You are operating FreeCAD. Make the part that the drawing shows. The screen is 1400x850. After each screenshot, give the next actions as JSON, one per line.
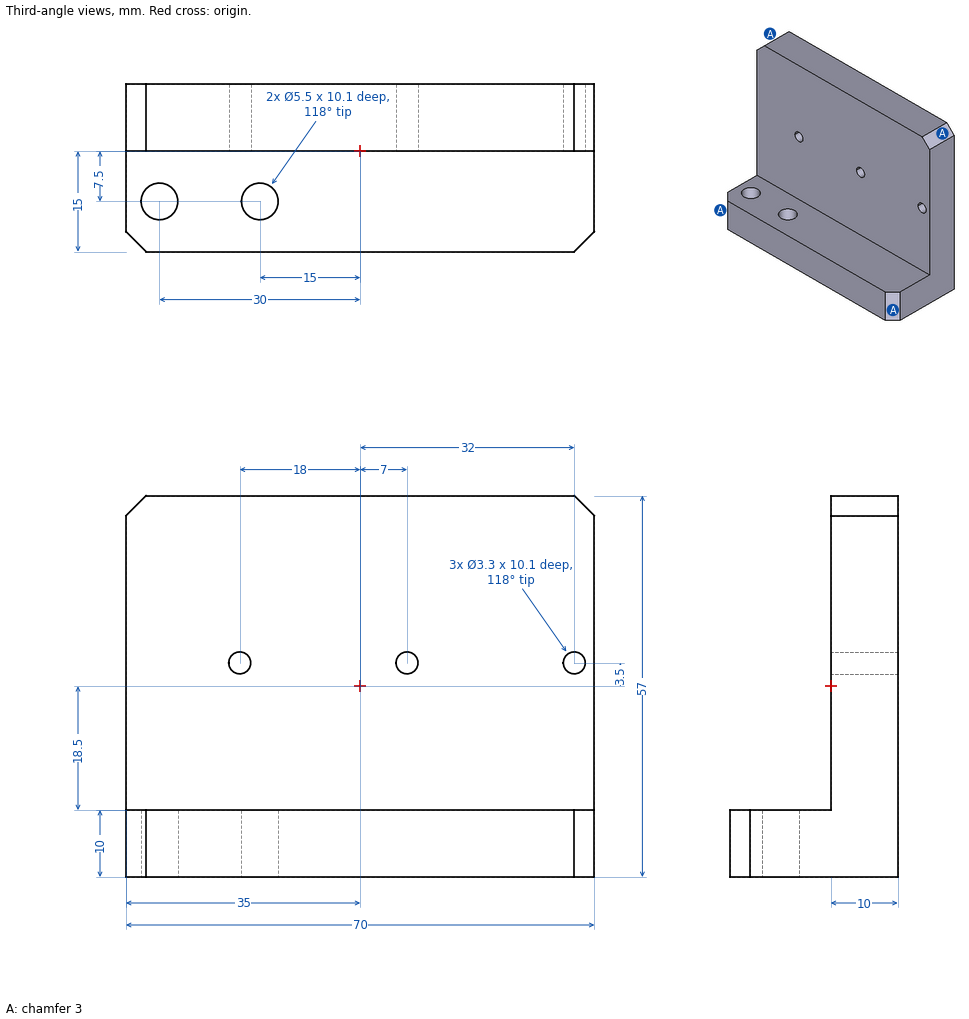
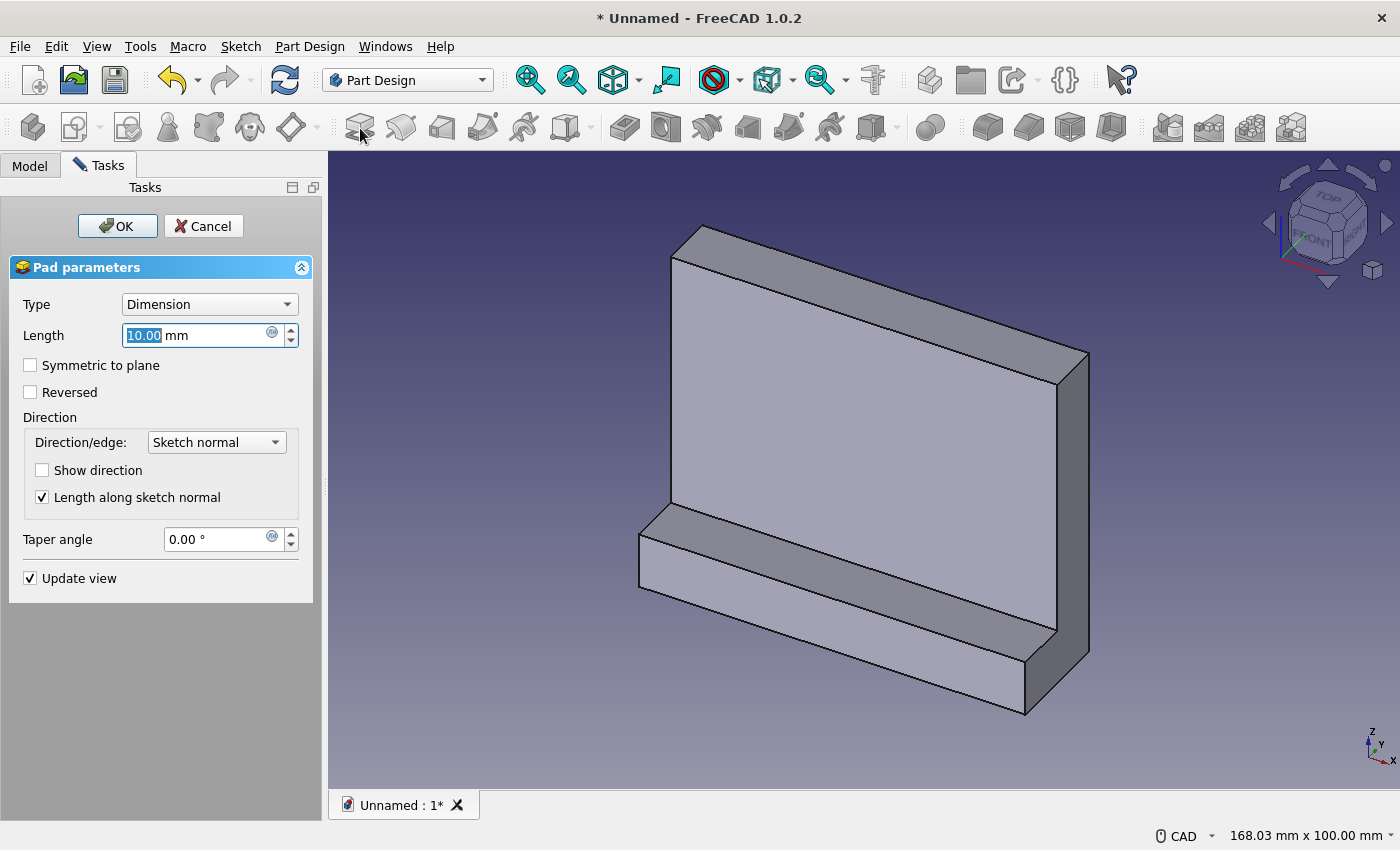
{"action": "type", "text": "15"}
{"action": "key", "text": "Tab"}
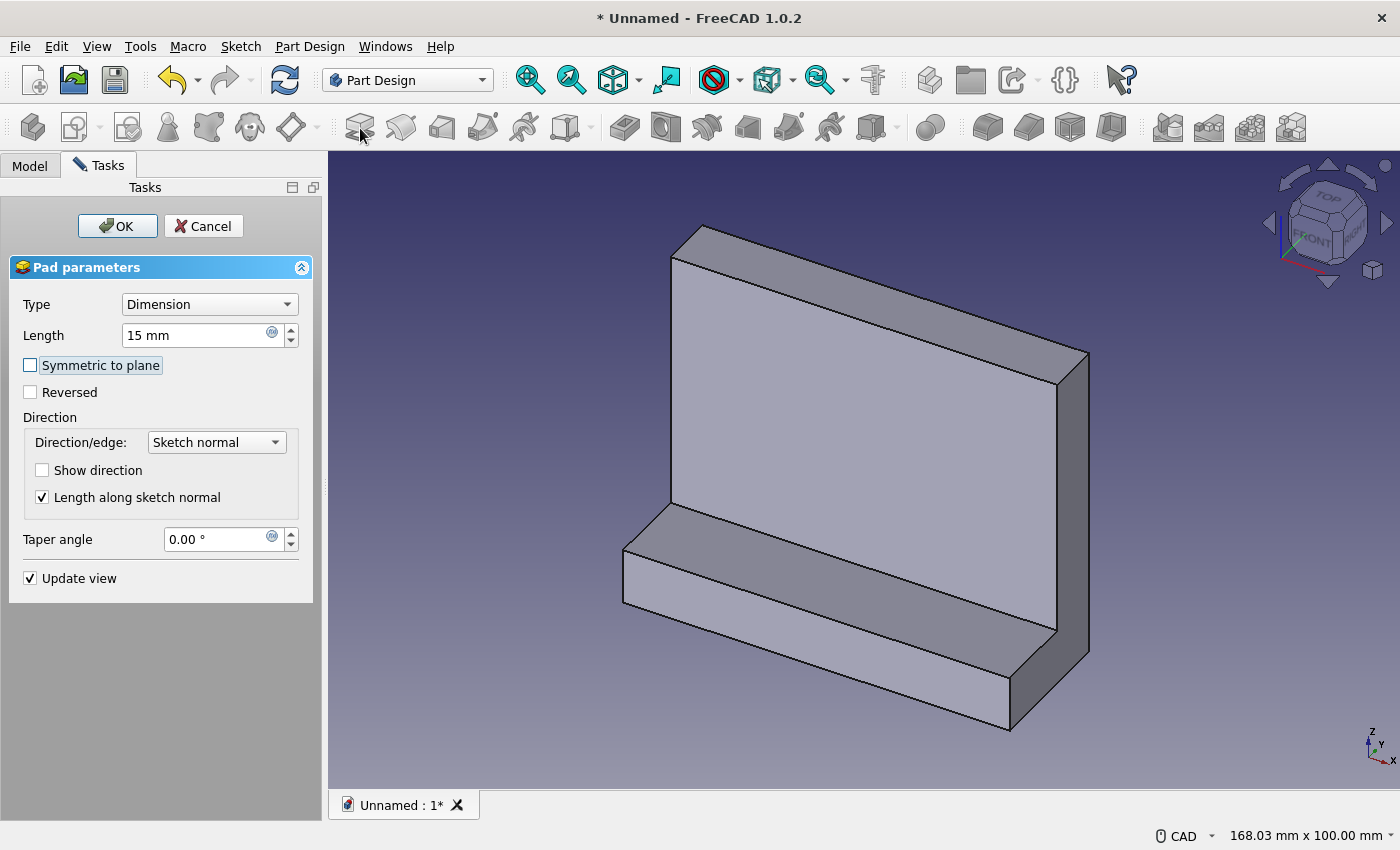
{"action": "left_click", "coordinate": [118, 226]}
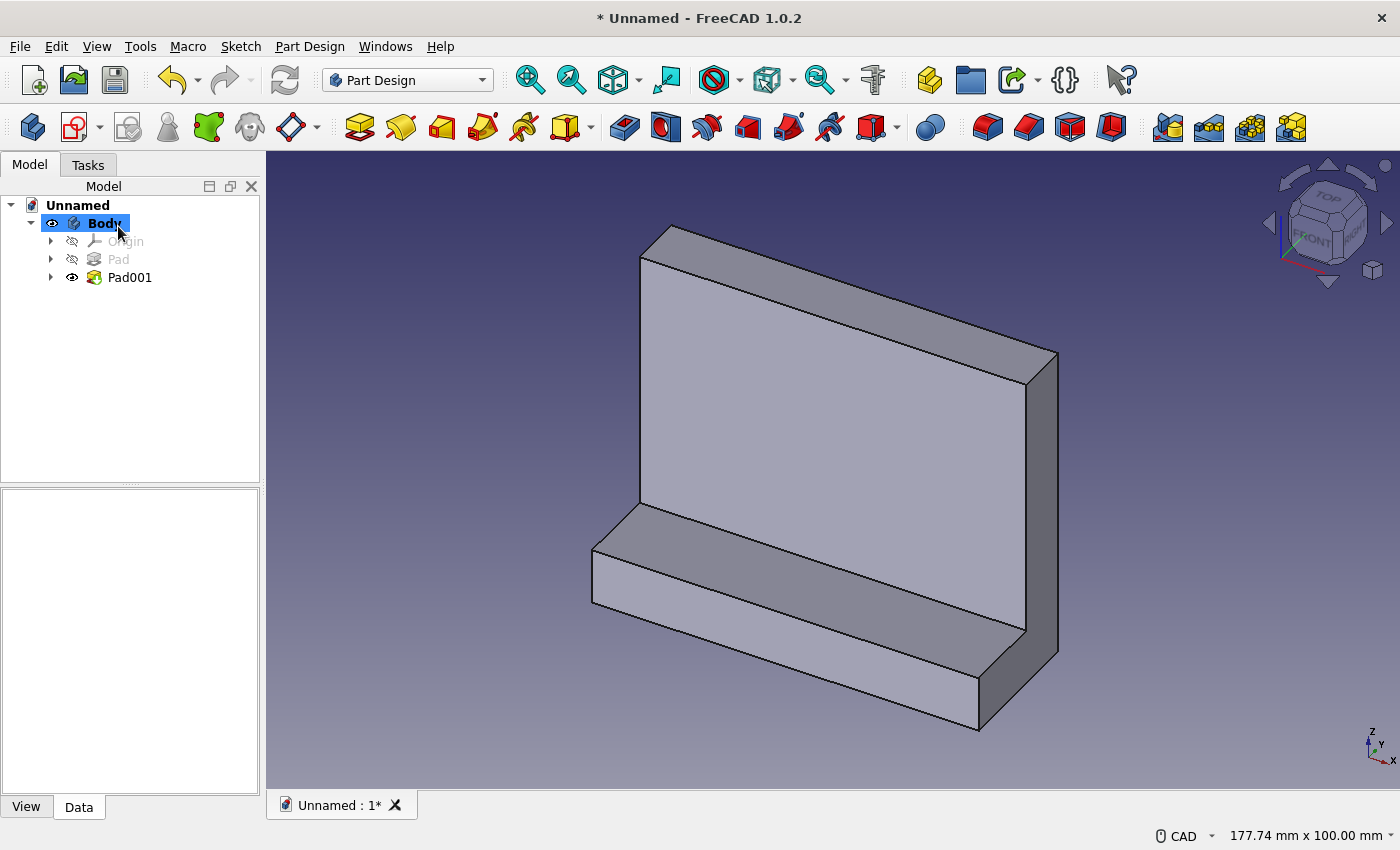
{"action": "left_click", "coordinate": [979, 703]}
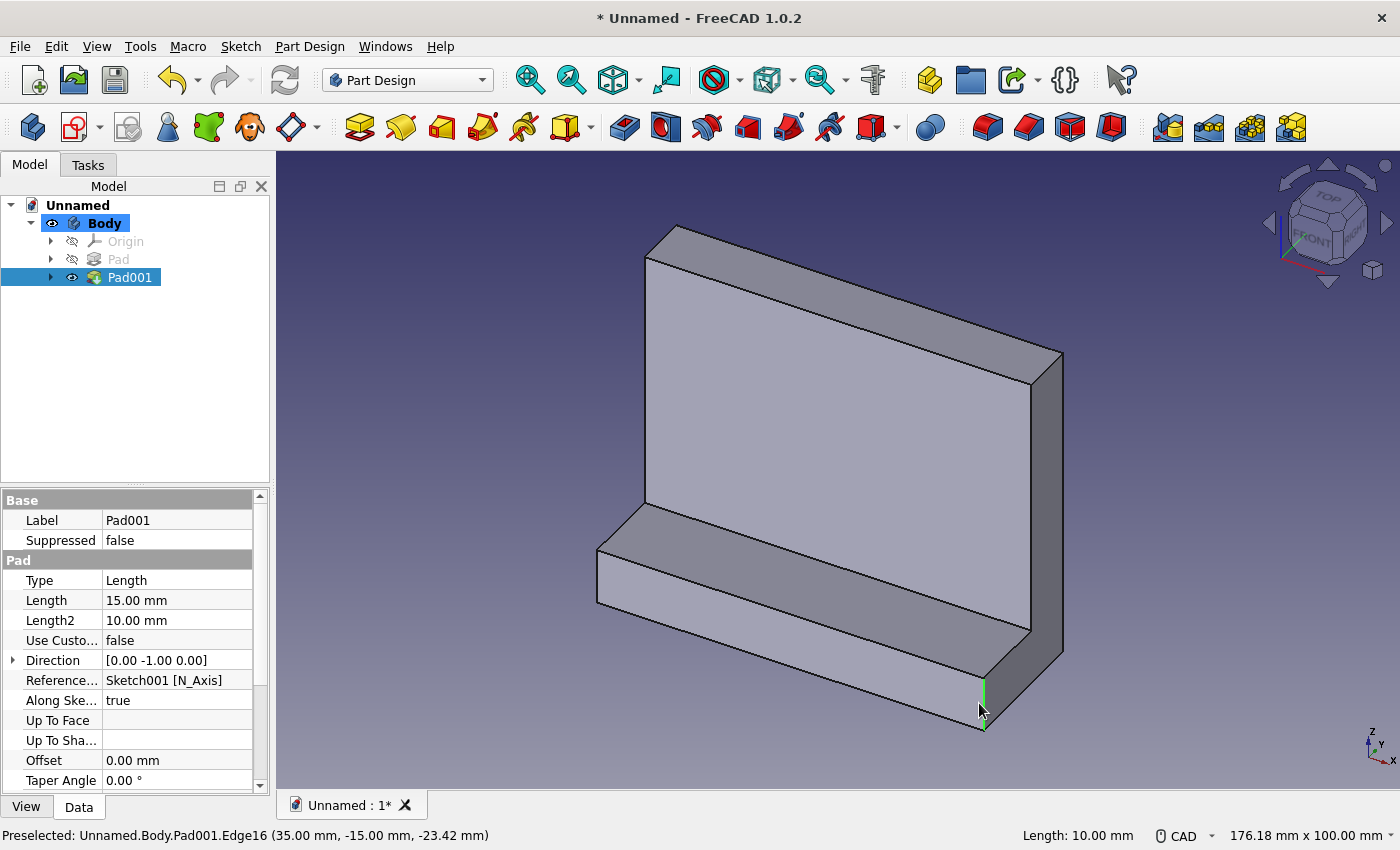
{"action": "left_click", "coordinate": [1047, 368], "text": "ctrl"}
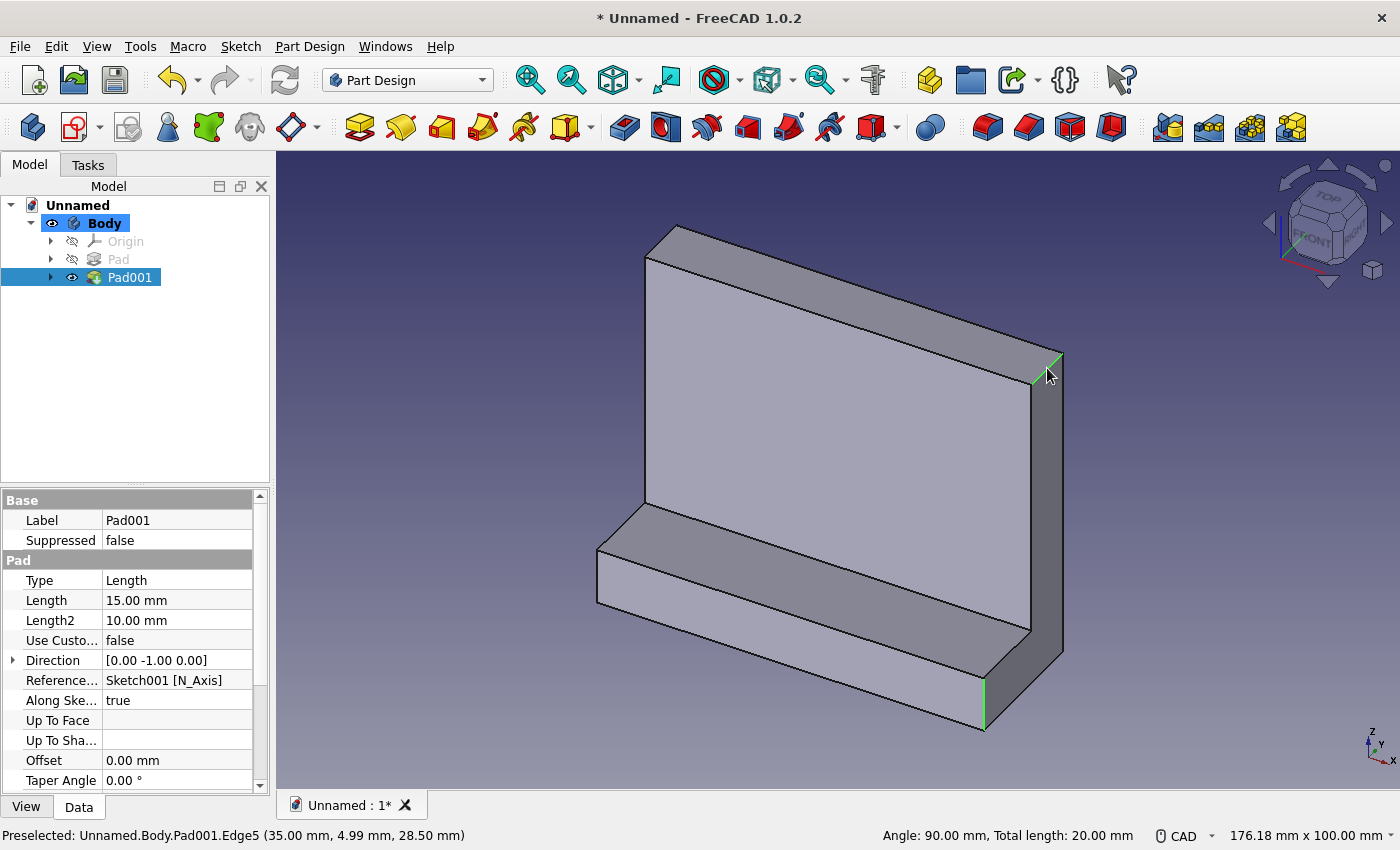
{"action": "key", "text": "0"}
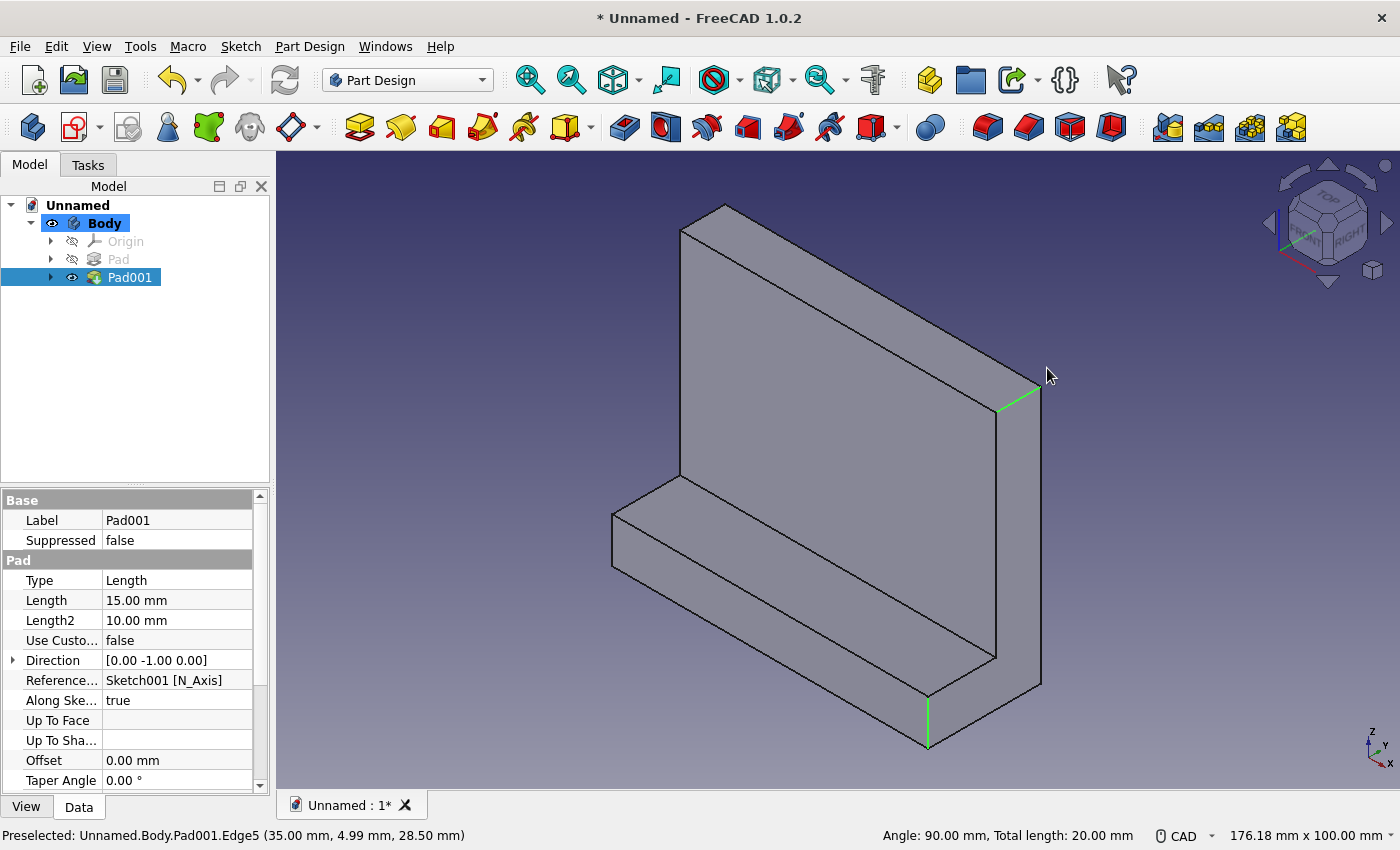
{"action": "key", "text": "2"}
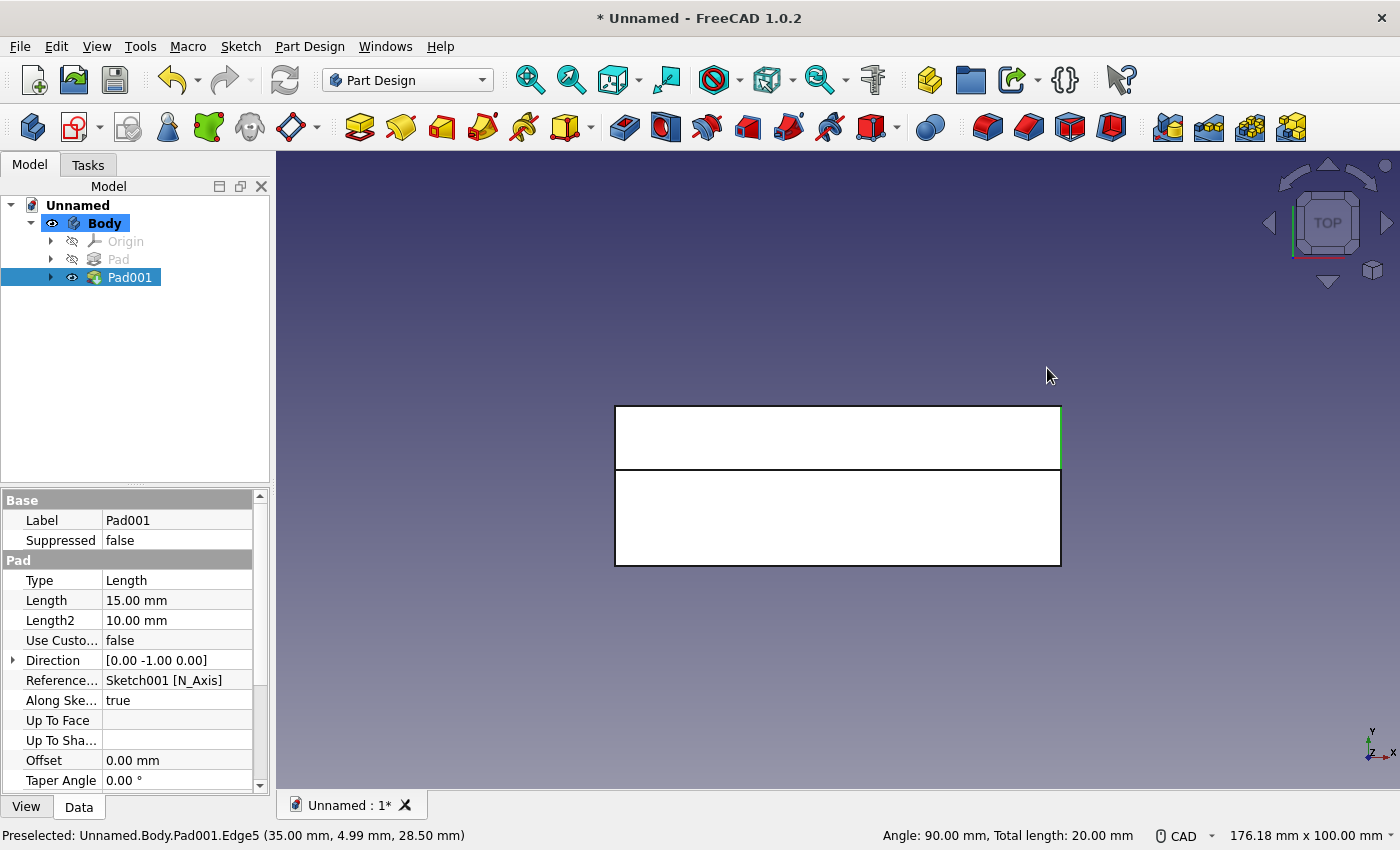
{"action": "left_click", "coordinate": [531, 80]}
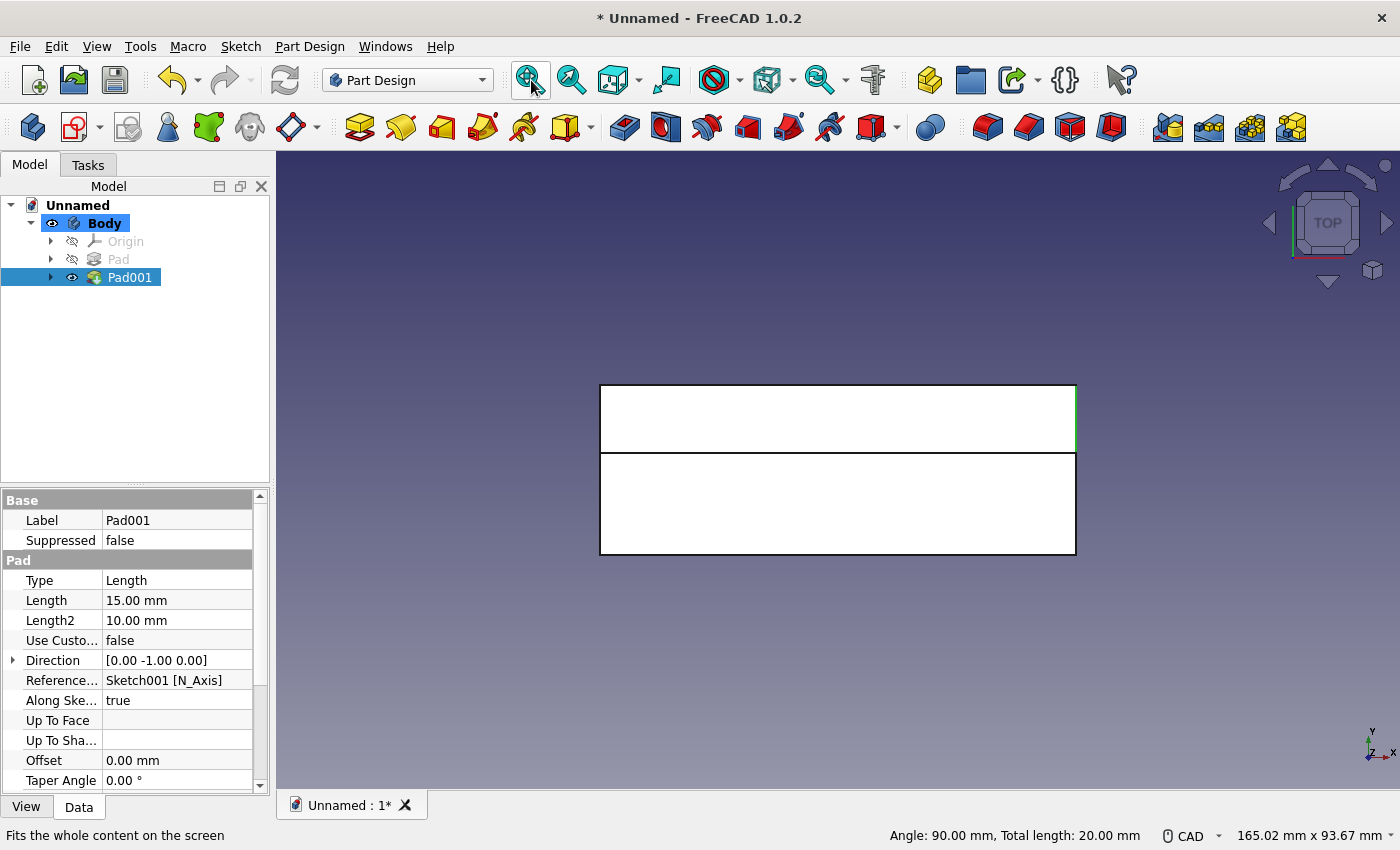
{"action": "left_click", "coordinate": [600, 418], "text": "ctrl"}